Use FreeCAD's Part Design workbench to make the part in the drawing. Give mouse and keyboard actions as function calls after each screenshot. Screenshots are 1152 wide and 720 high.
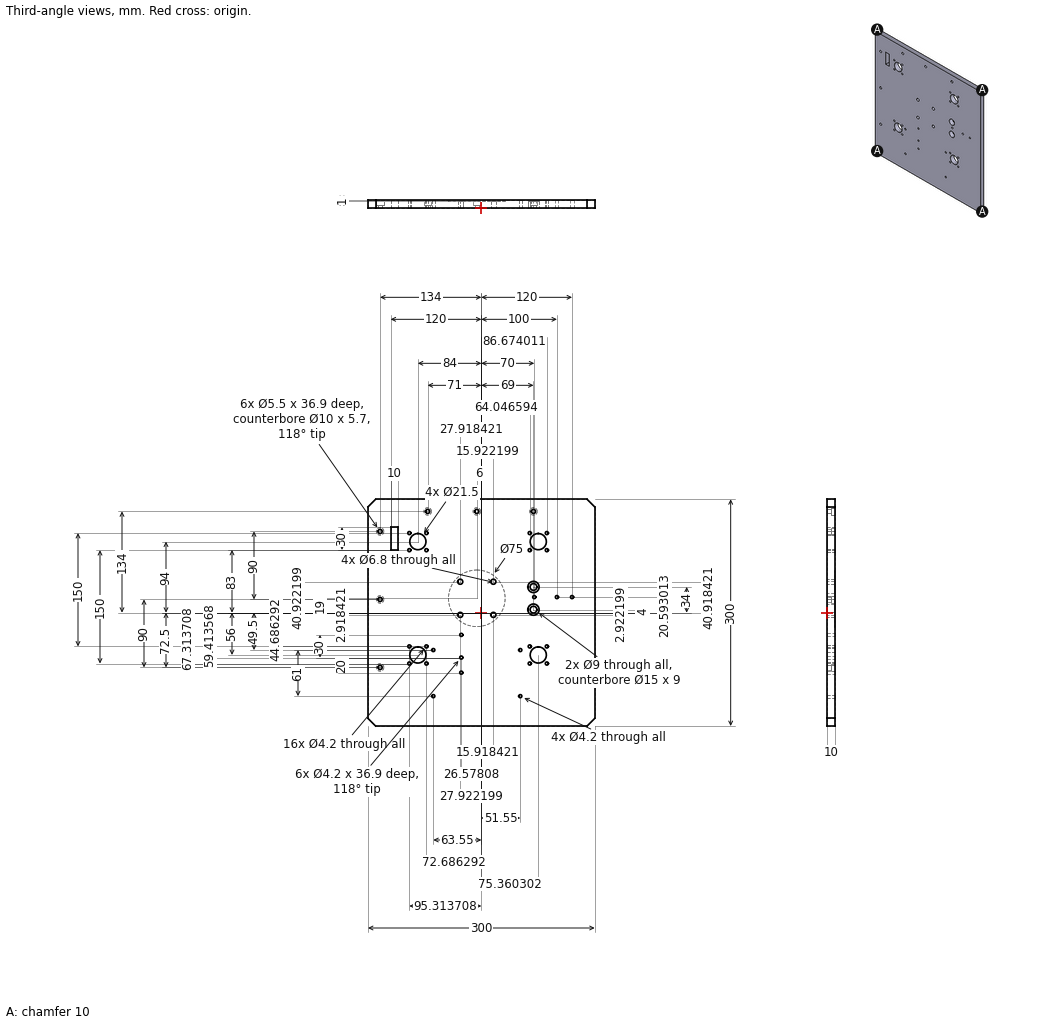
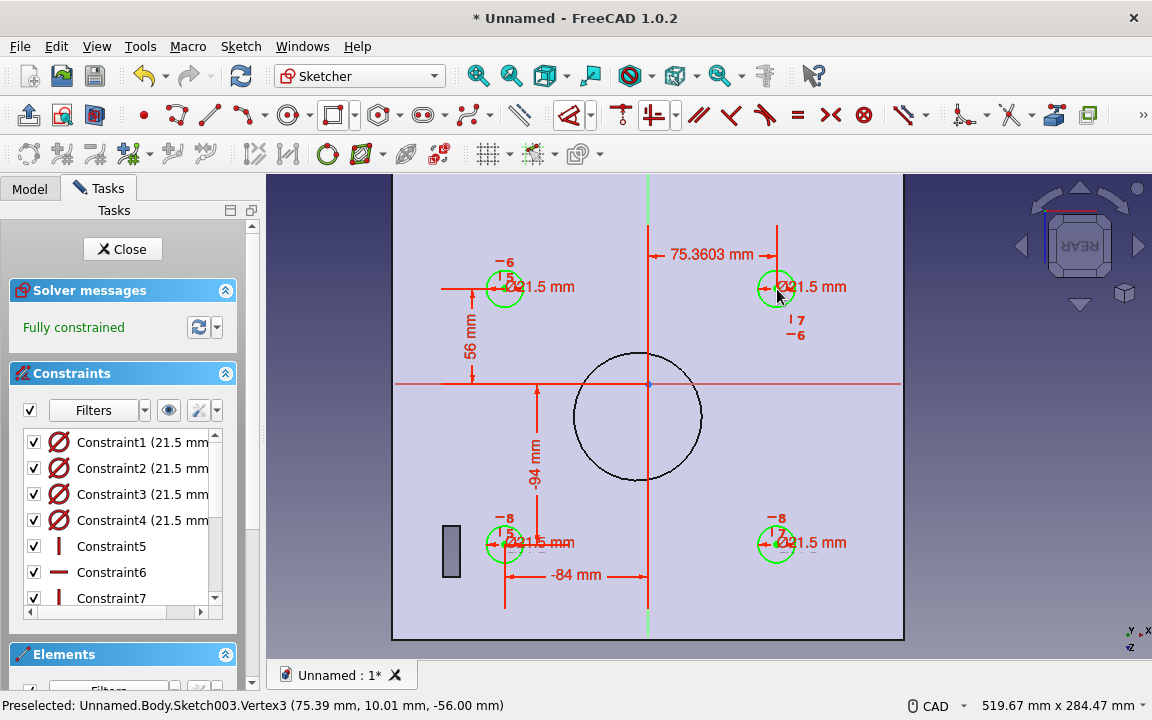
click(123, 249)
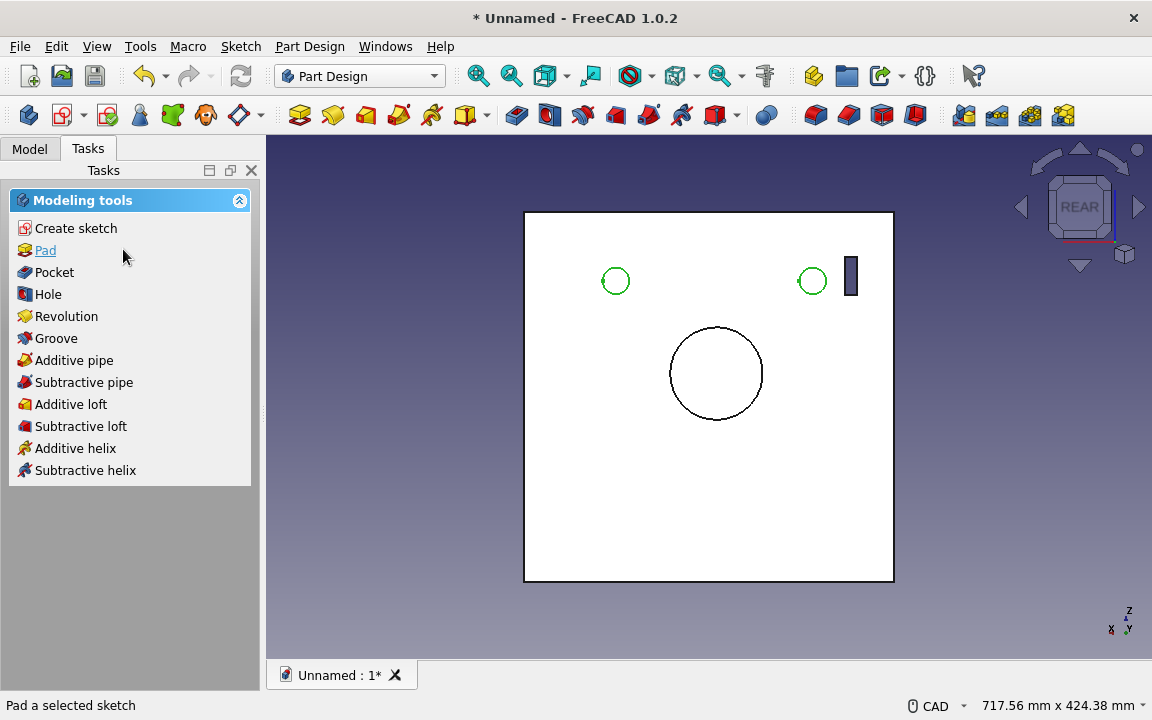
click(517, 116)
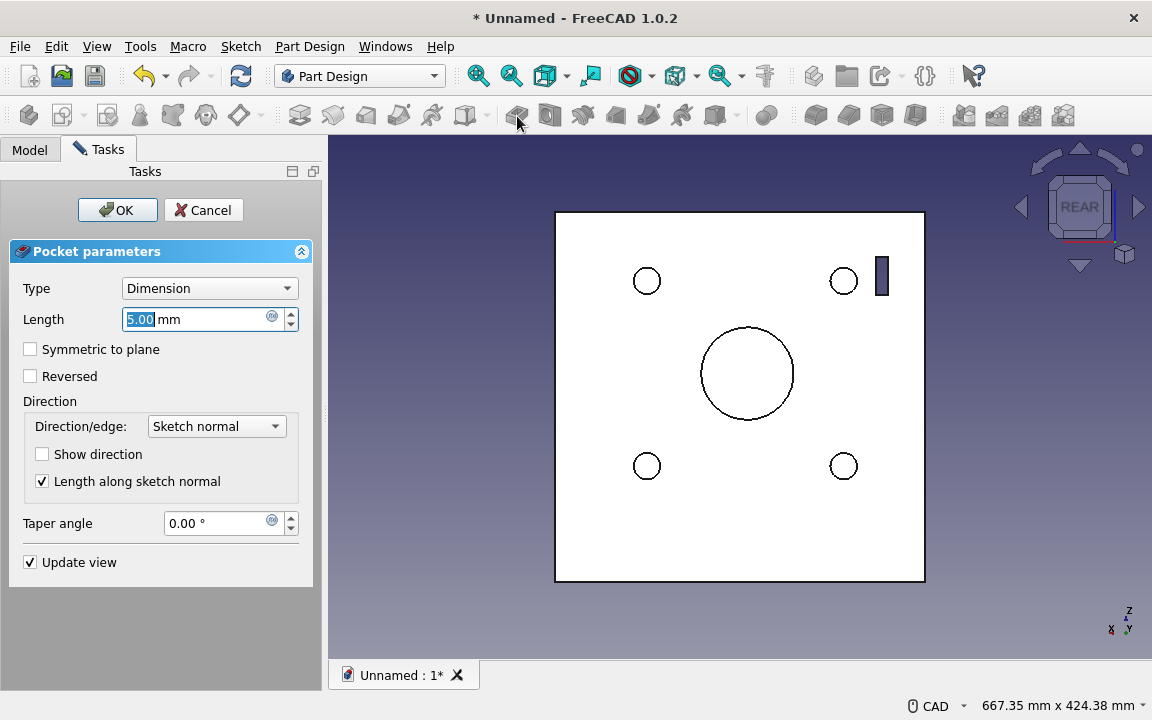
click(210, 288)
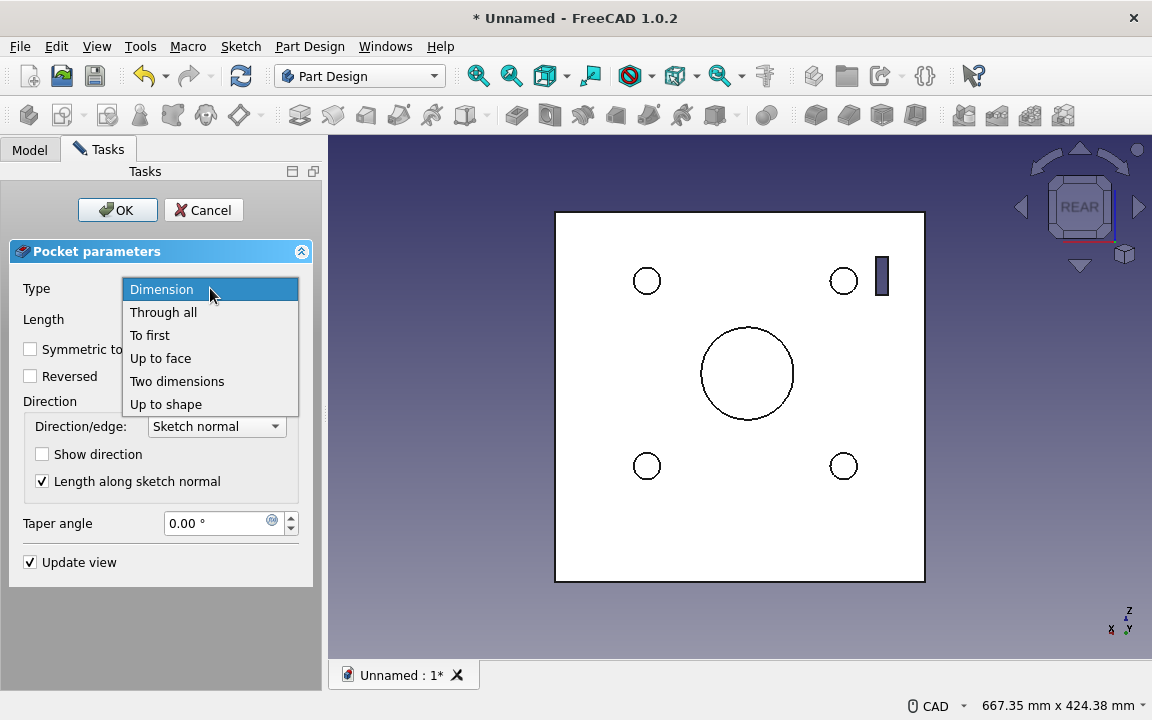
click(208, 312)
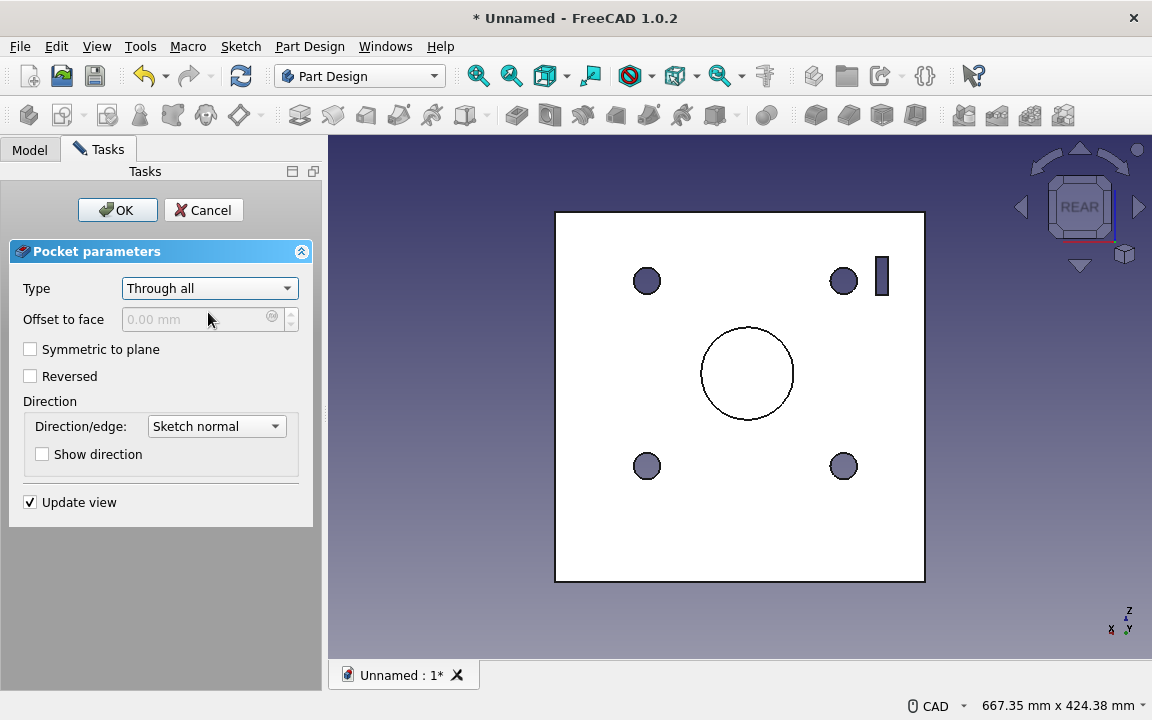
click(118, 210)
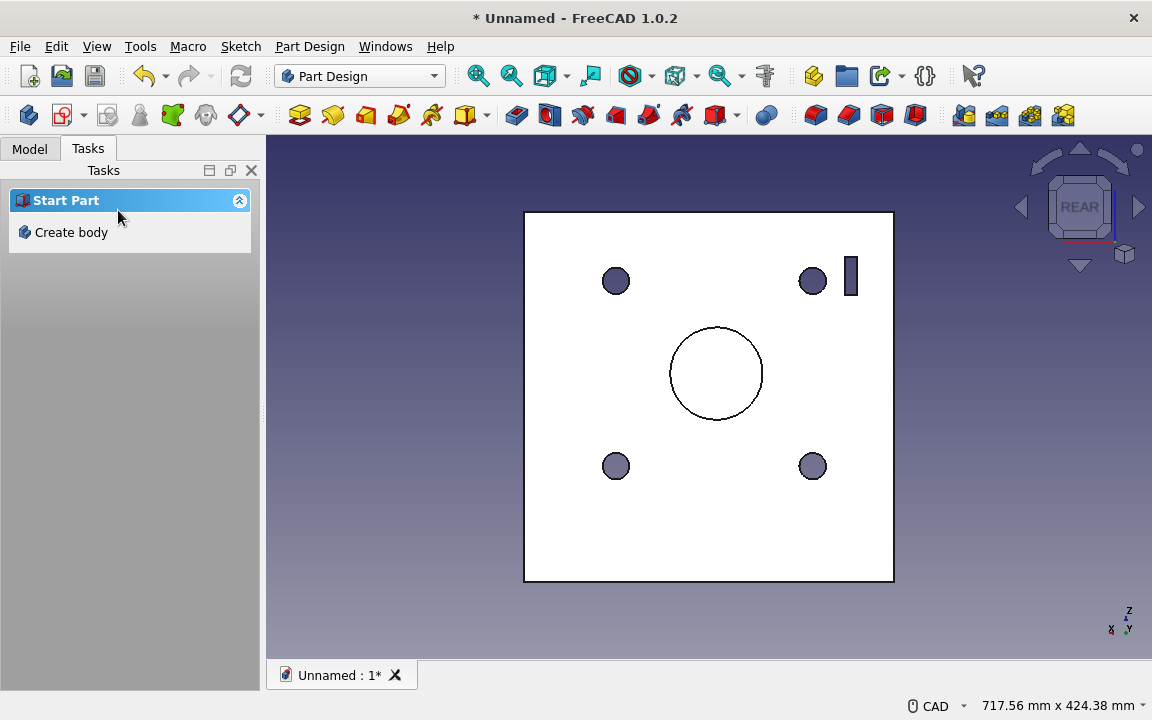
key(0)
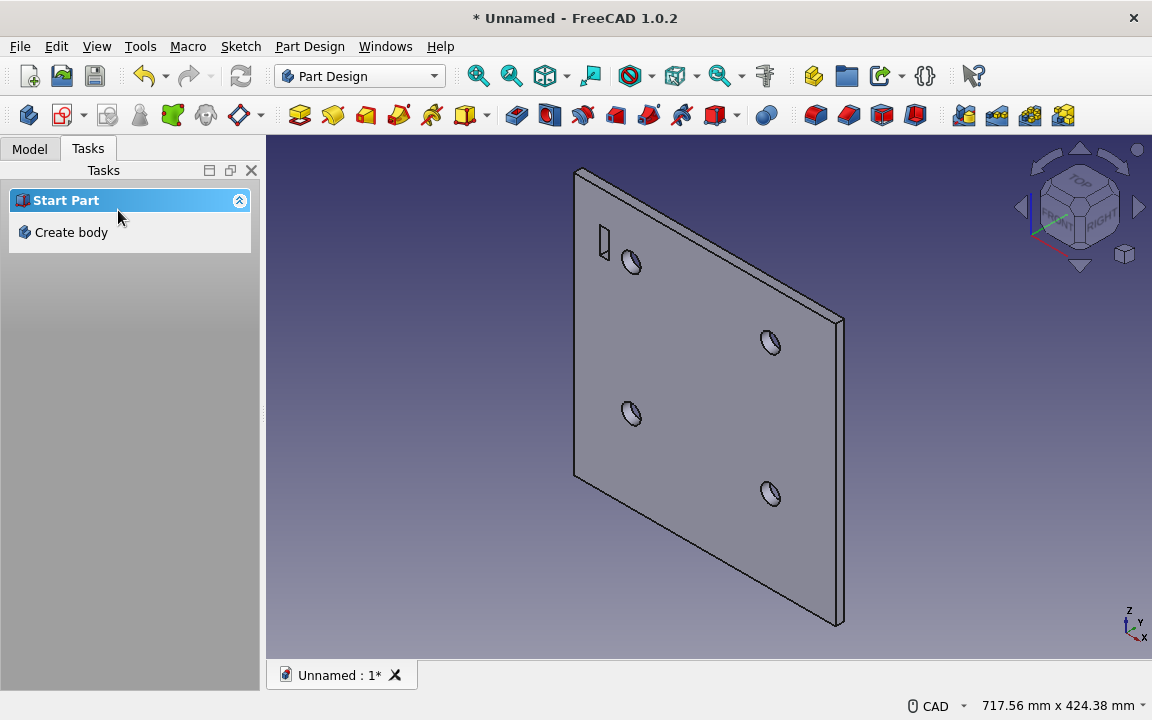
click(705, 399)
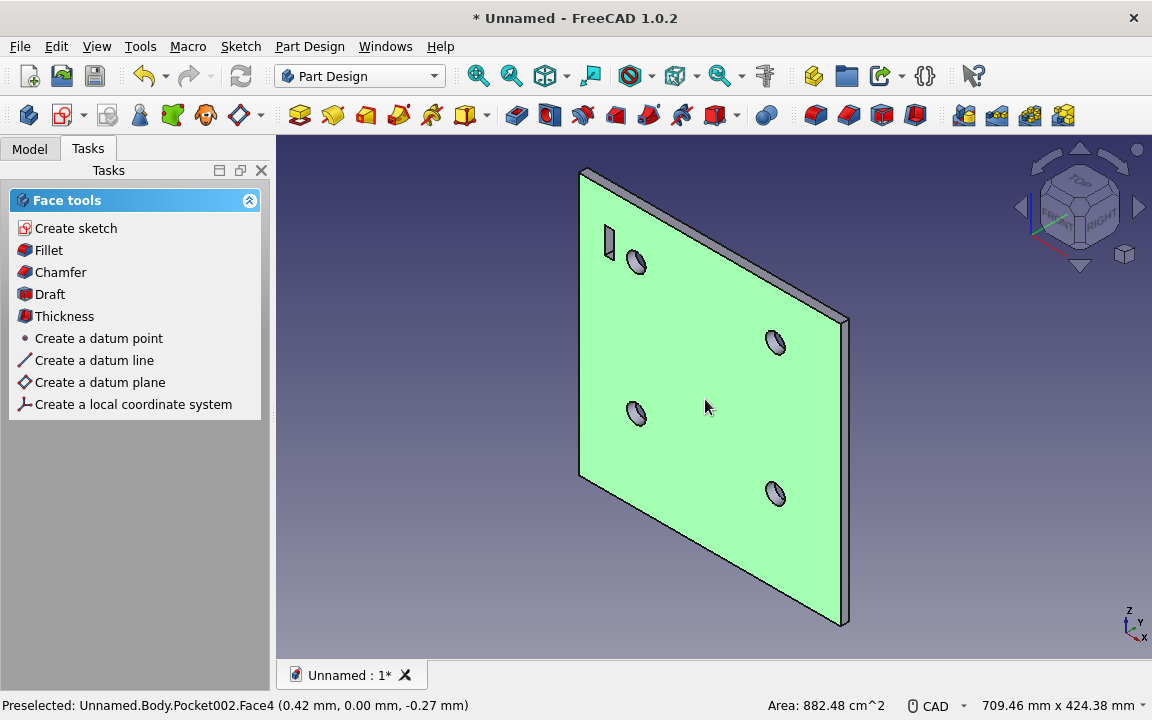
click(62, 116)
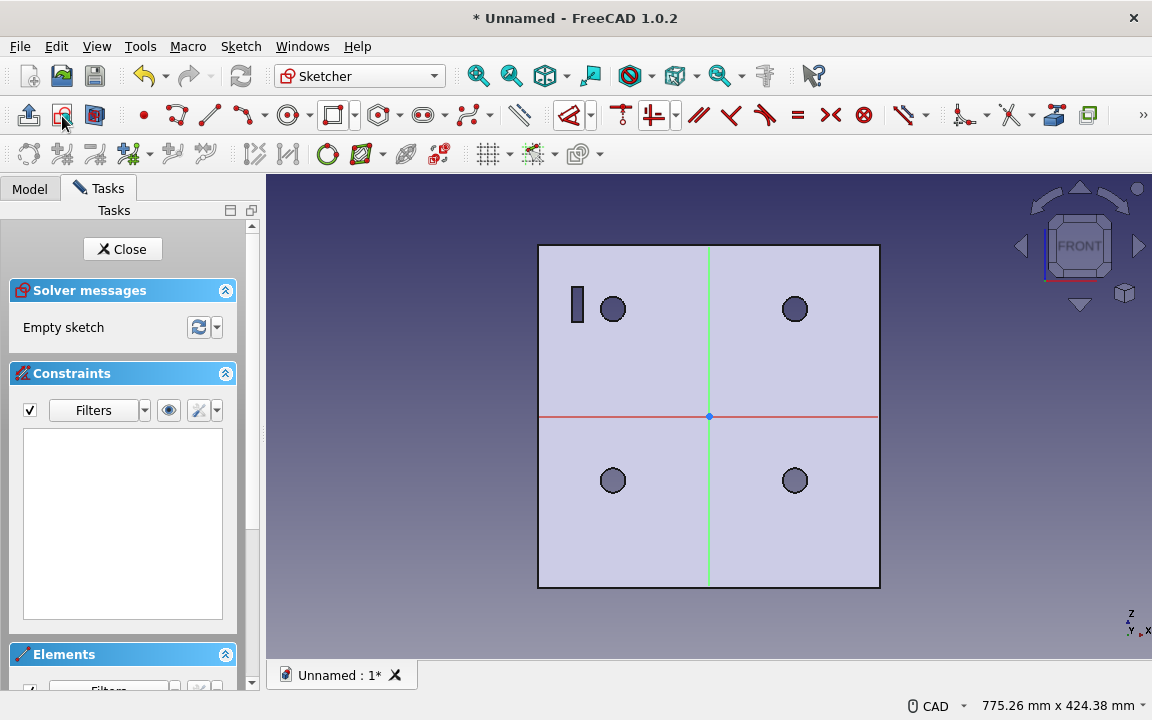
scroll(773, 390, up, 9)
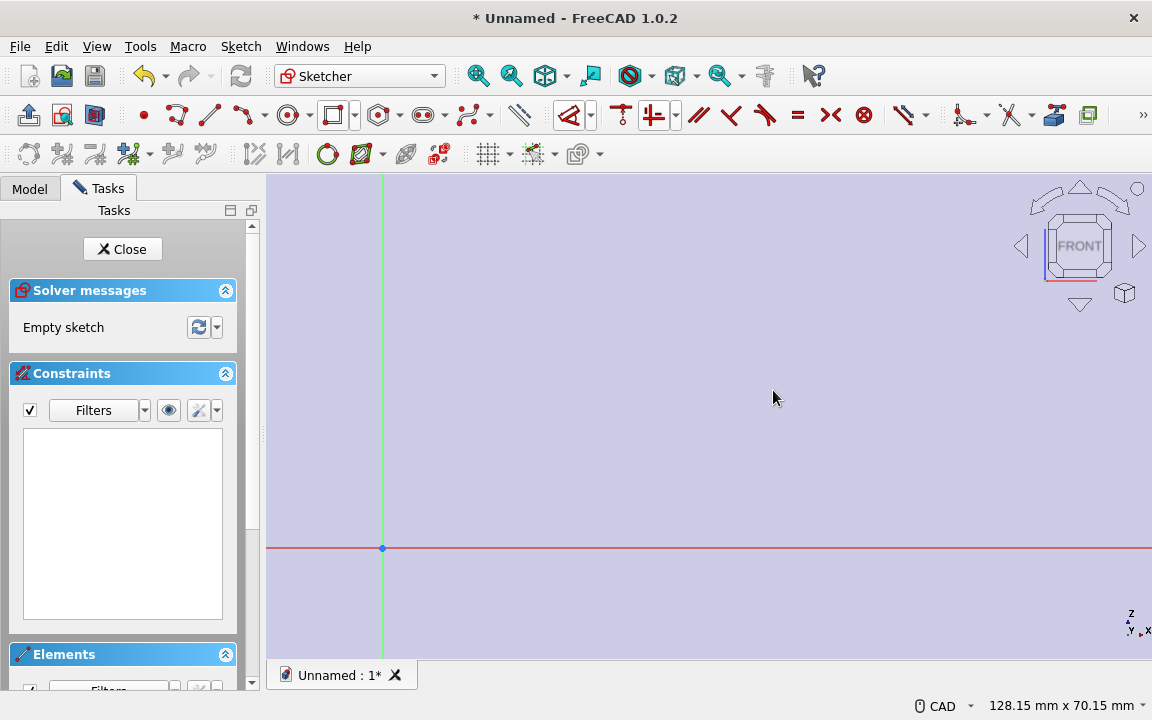
click(288, 116)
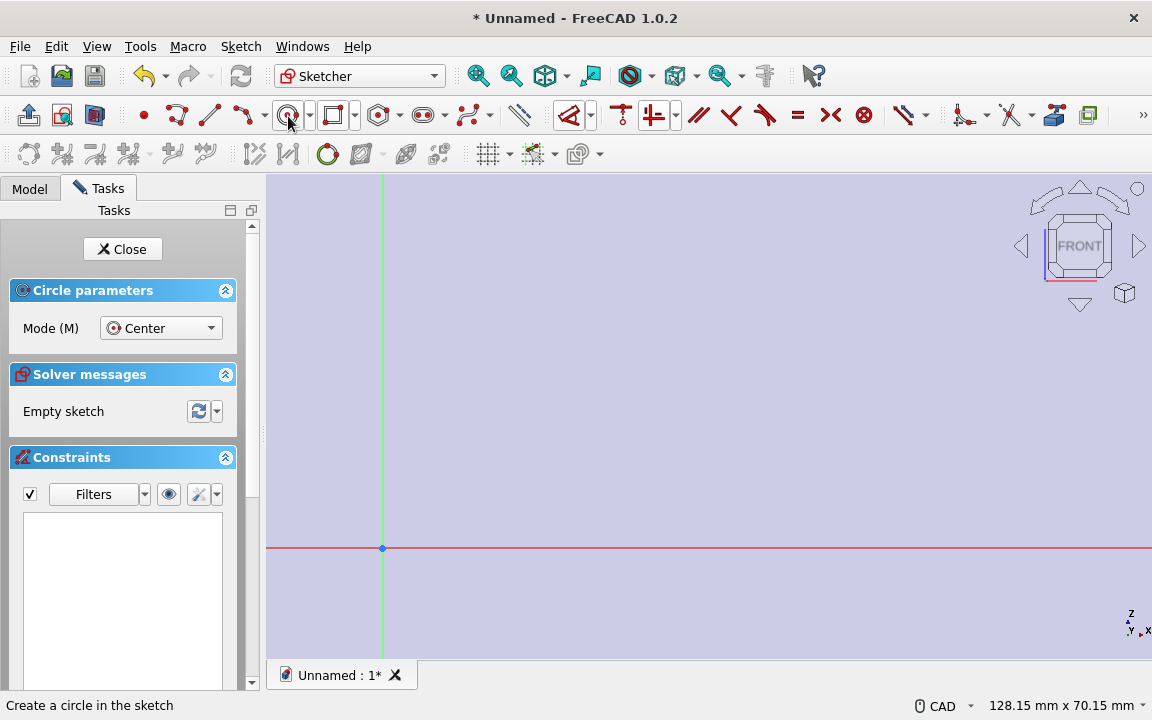
click(860, 520)
move(882, 498)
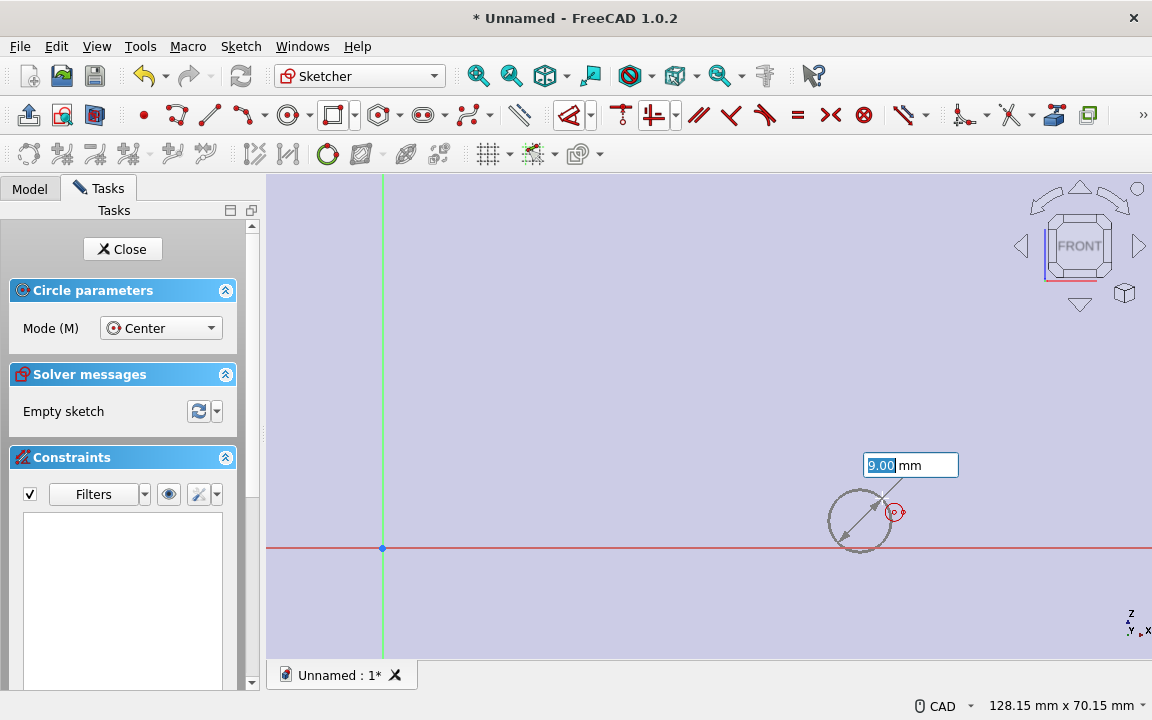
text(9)
key(Return)